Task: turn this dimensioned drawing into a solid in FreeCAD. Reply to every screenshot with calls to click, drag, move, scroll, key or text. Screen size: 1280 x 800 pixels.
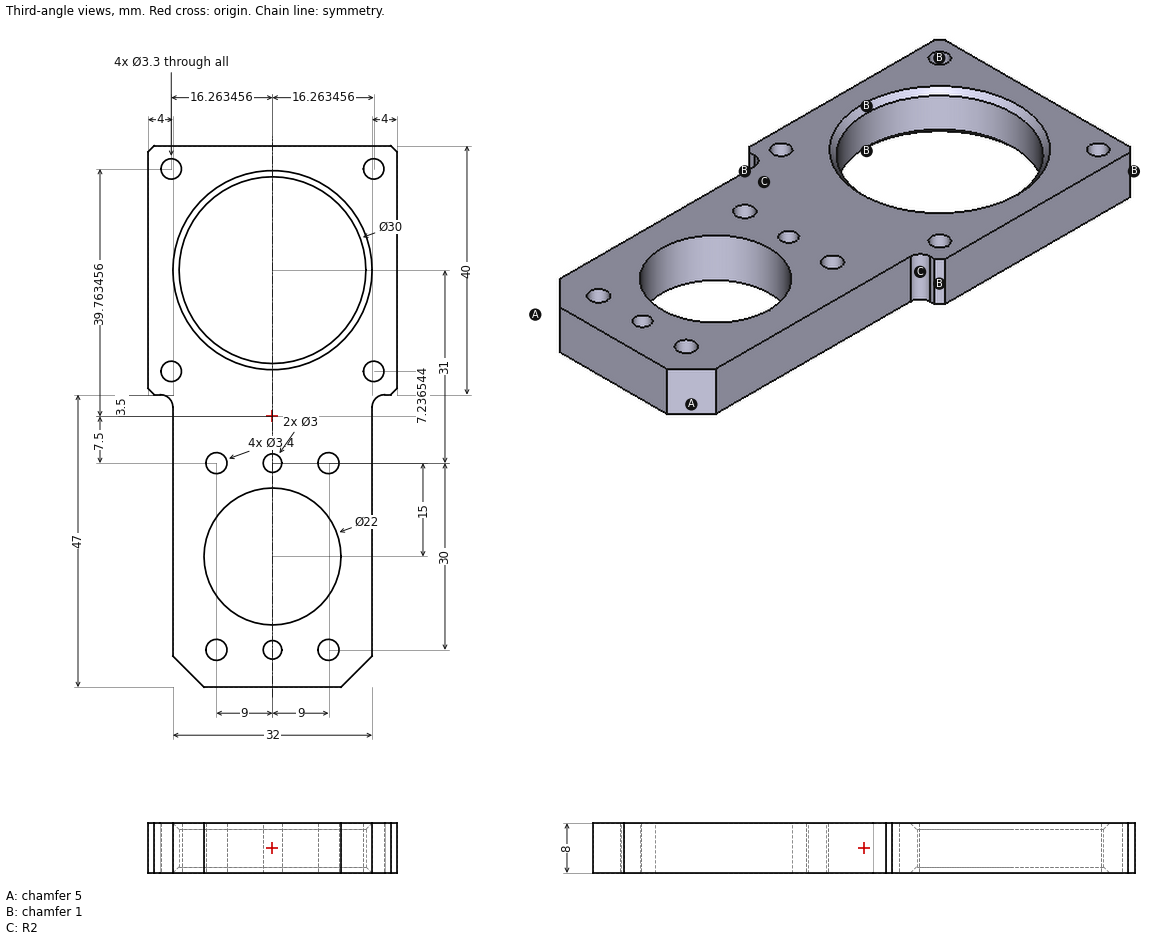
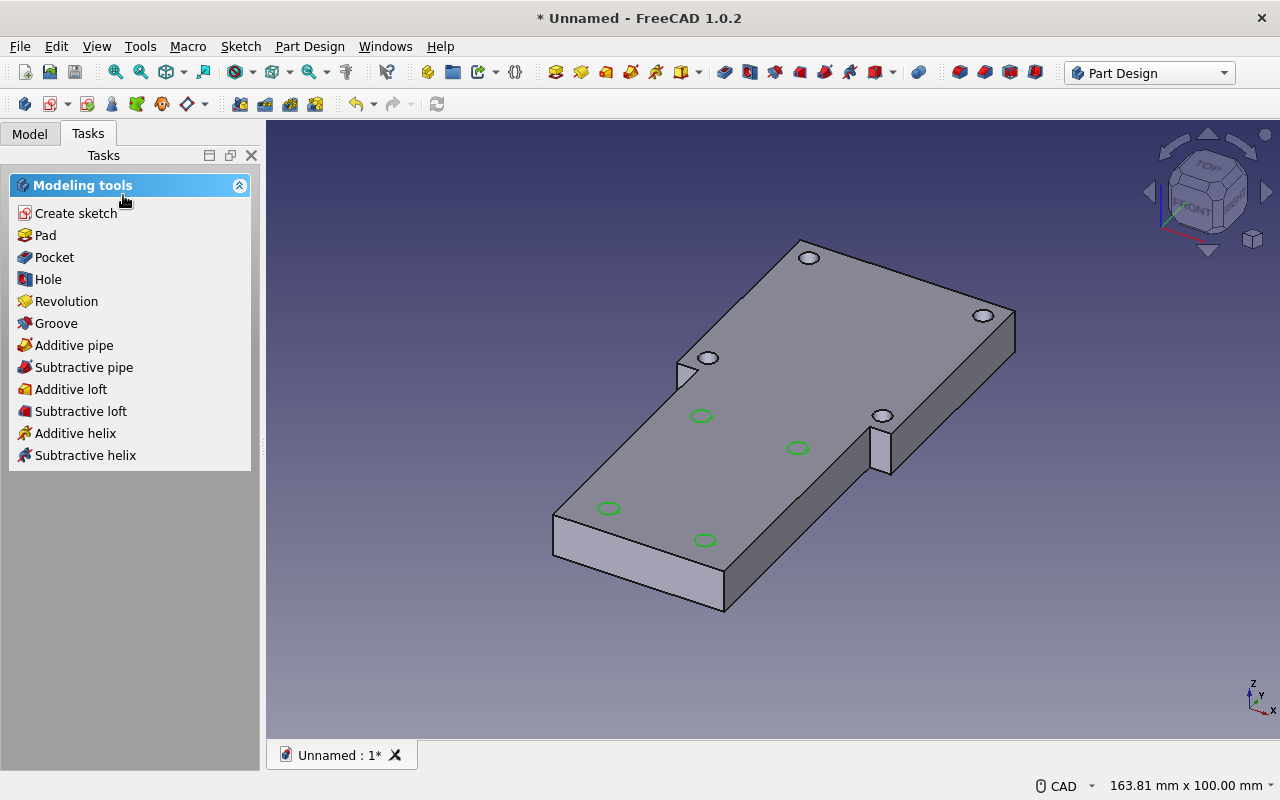
click(725, 72)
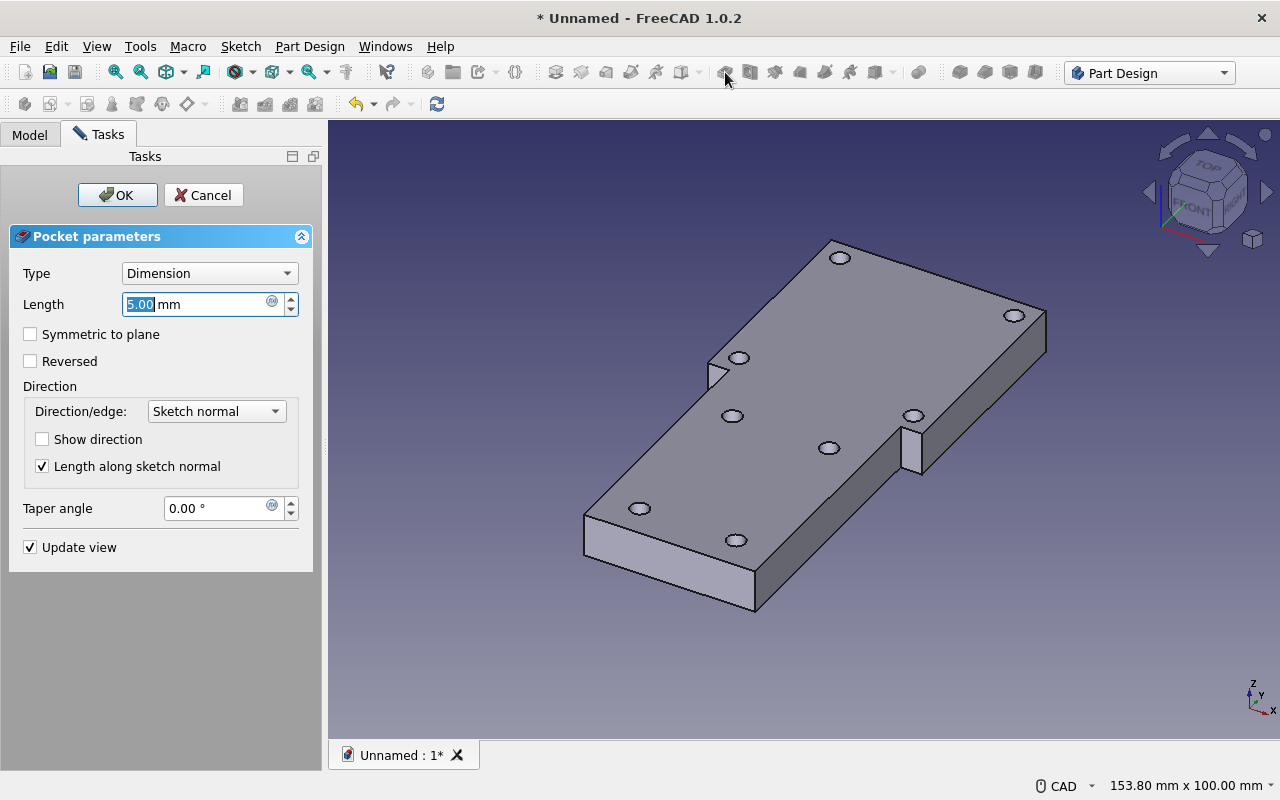
click(210, 274)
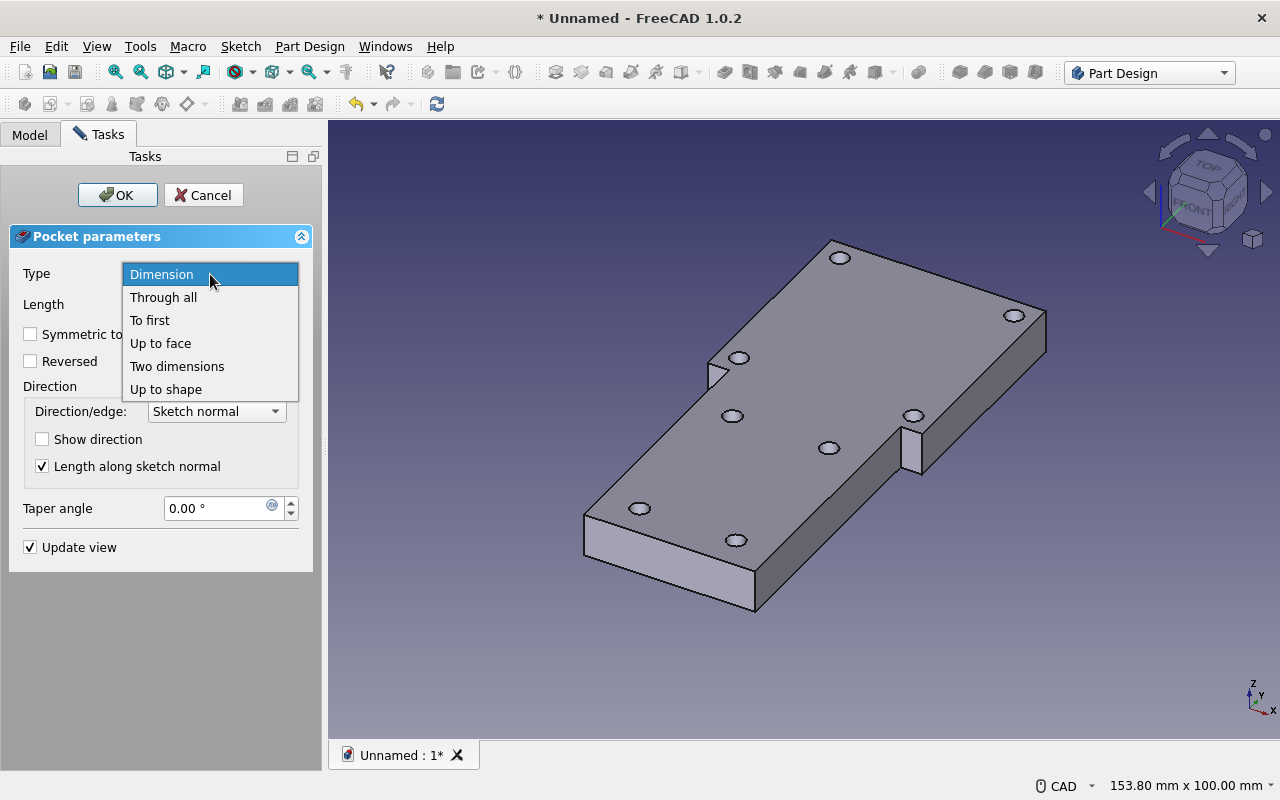
click(208, 298)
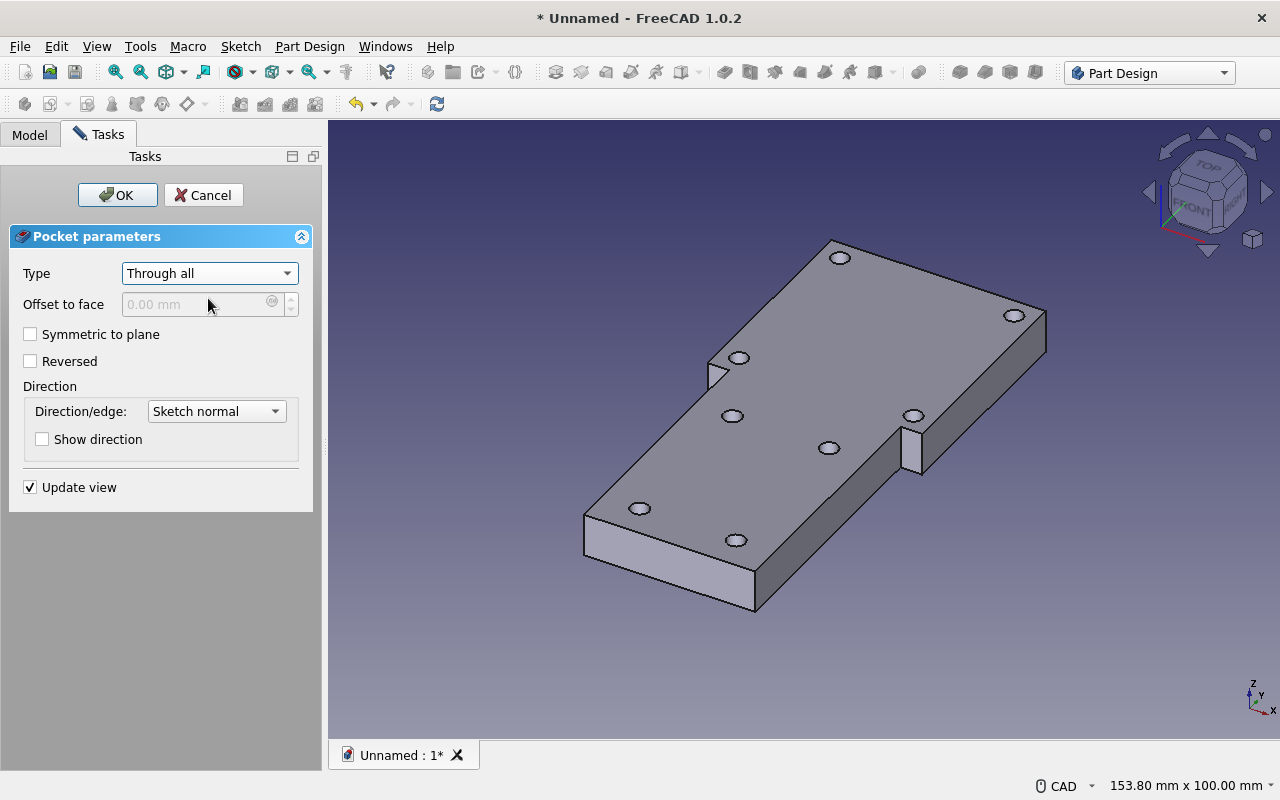
click(118, 195)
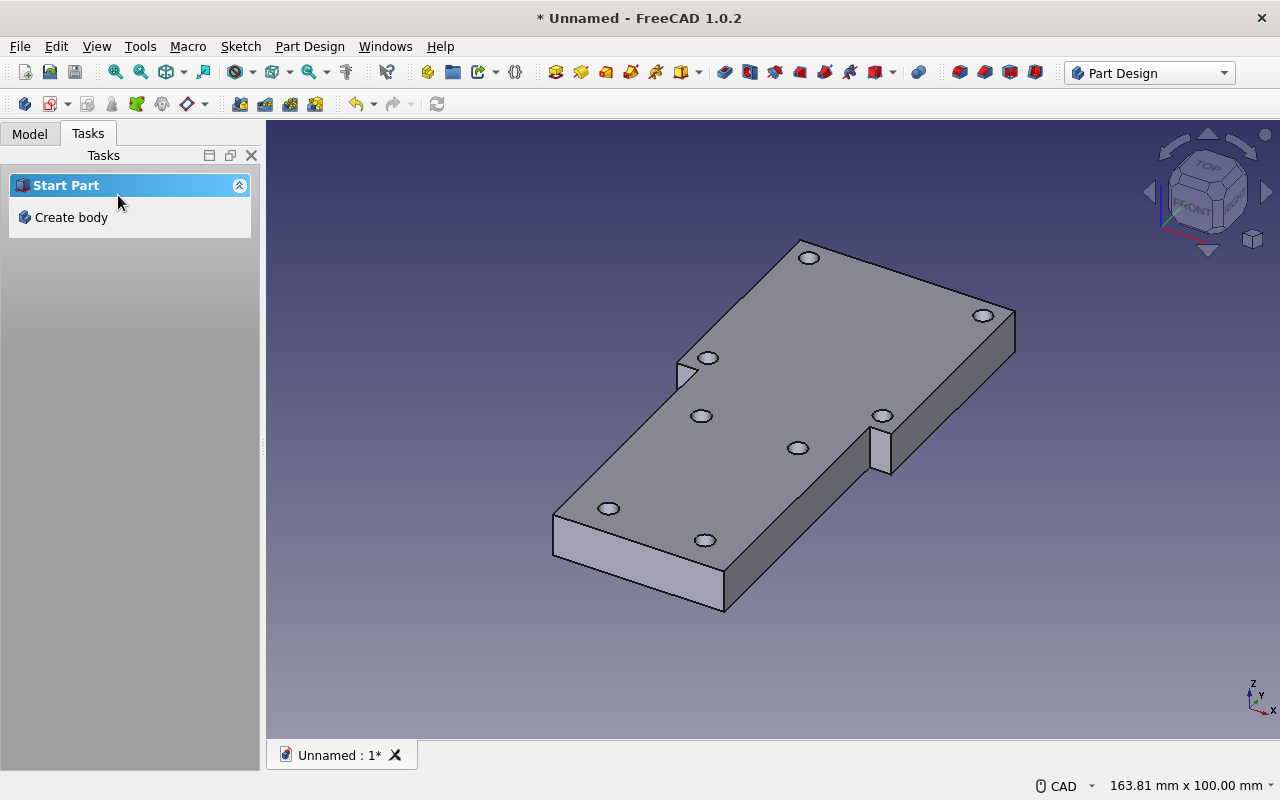
click(850, 332)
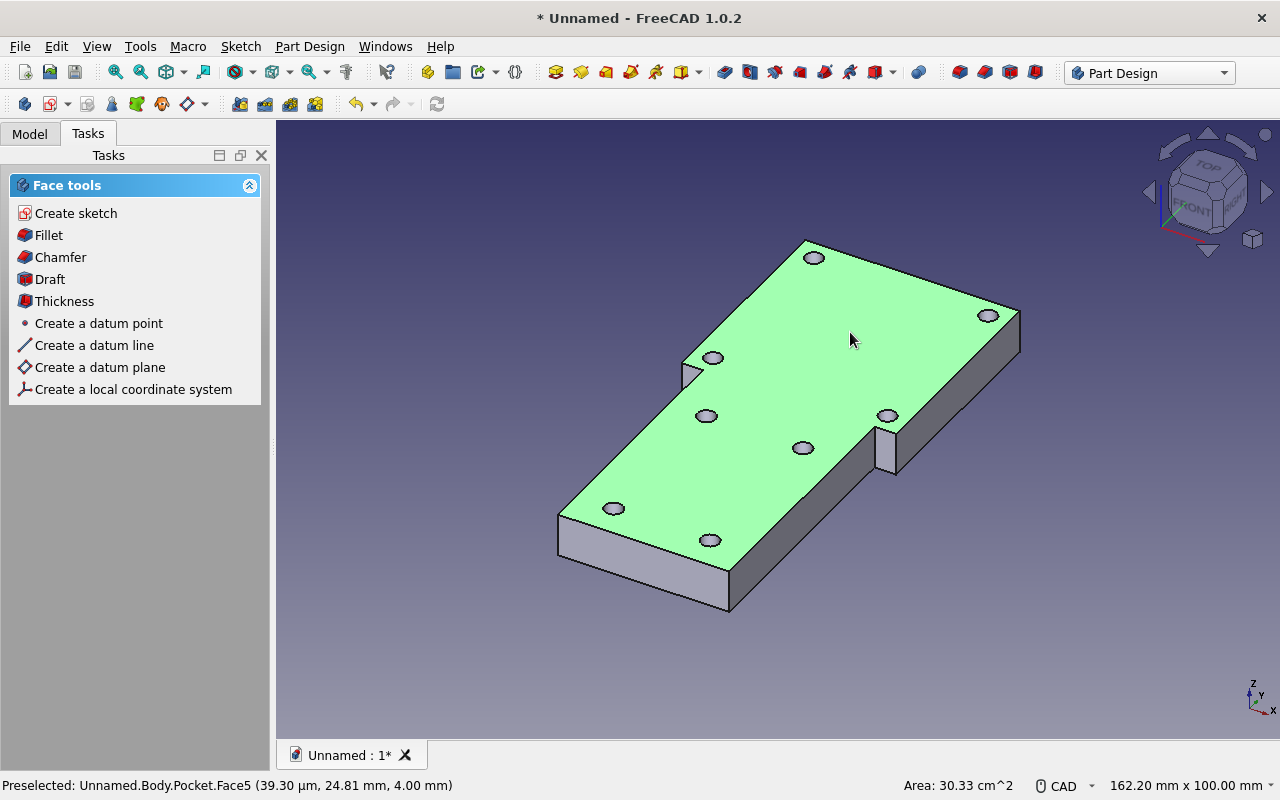
click(50, 104)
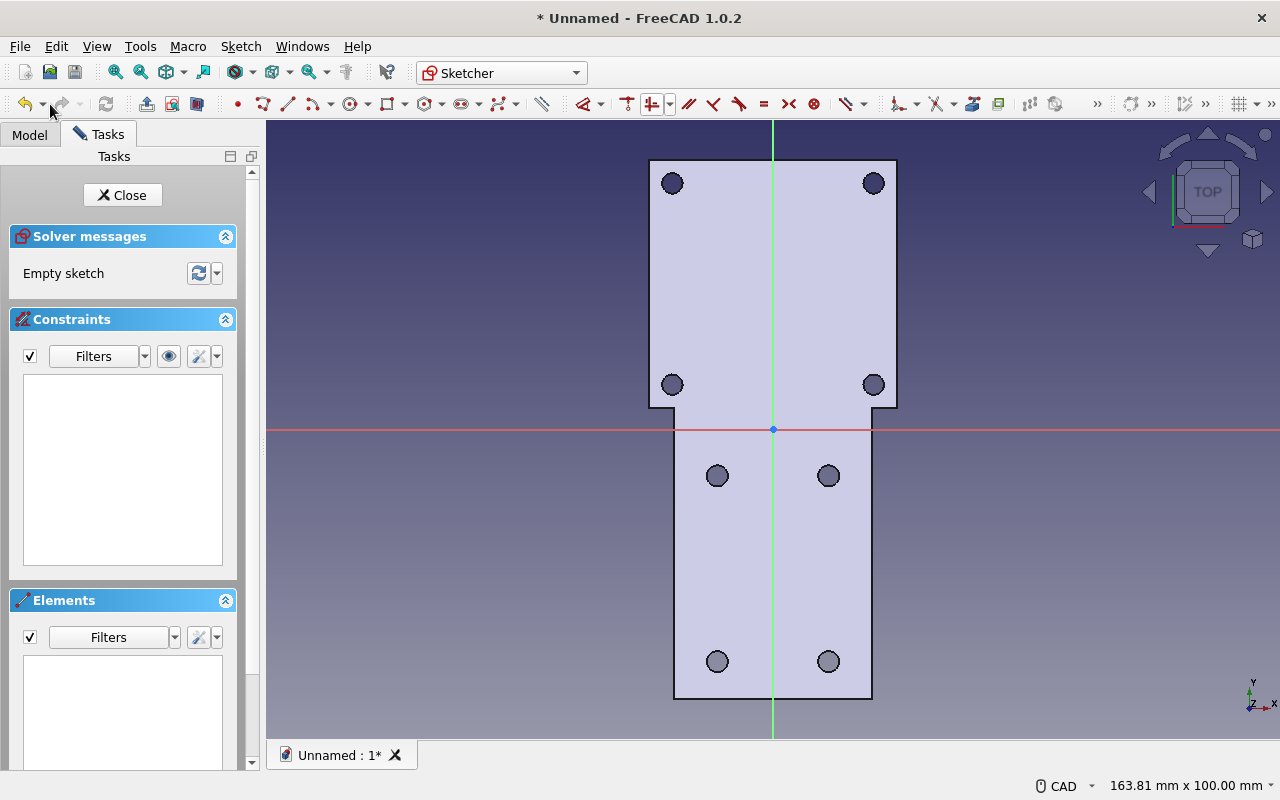
key(g)
key(c)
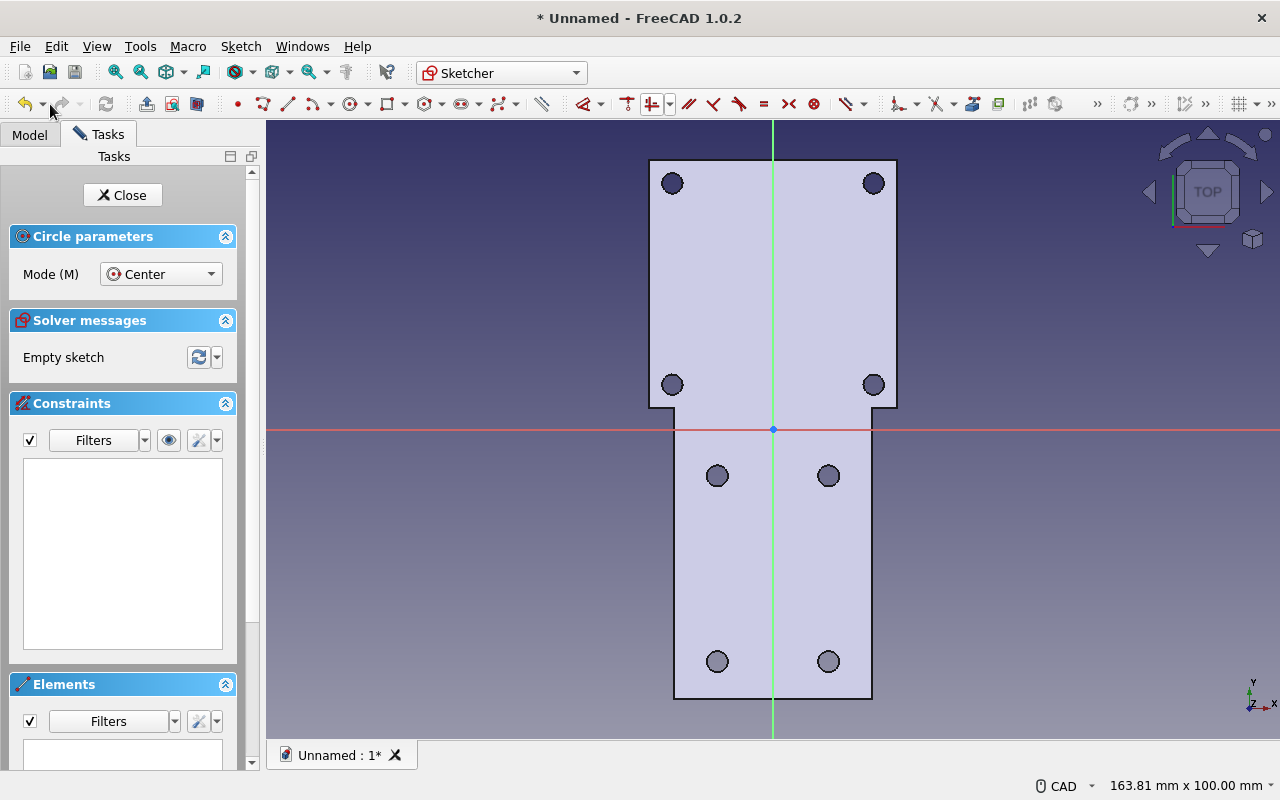
click(773, 284)
click(839, 218)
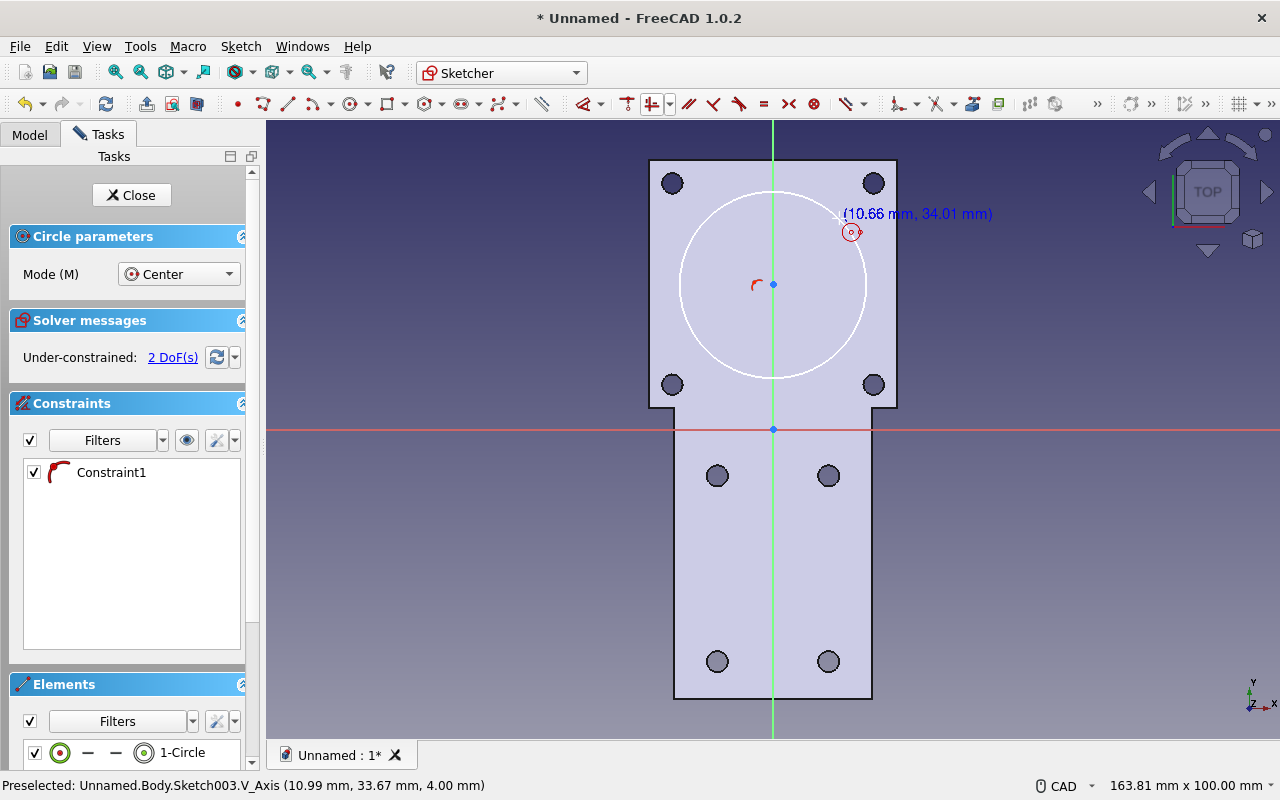
scroll(773, 476, up, 5)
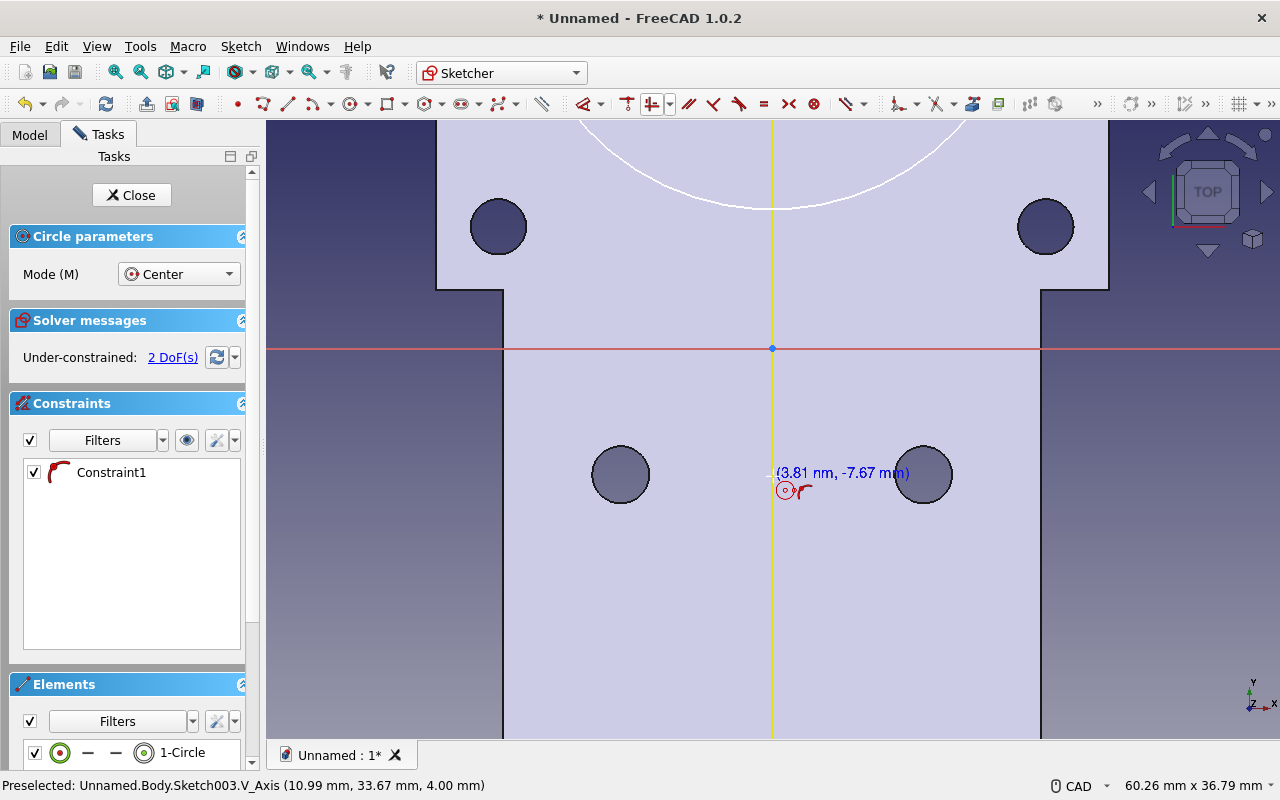
click(772, 475)
click(790, 457)